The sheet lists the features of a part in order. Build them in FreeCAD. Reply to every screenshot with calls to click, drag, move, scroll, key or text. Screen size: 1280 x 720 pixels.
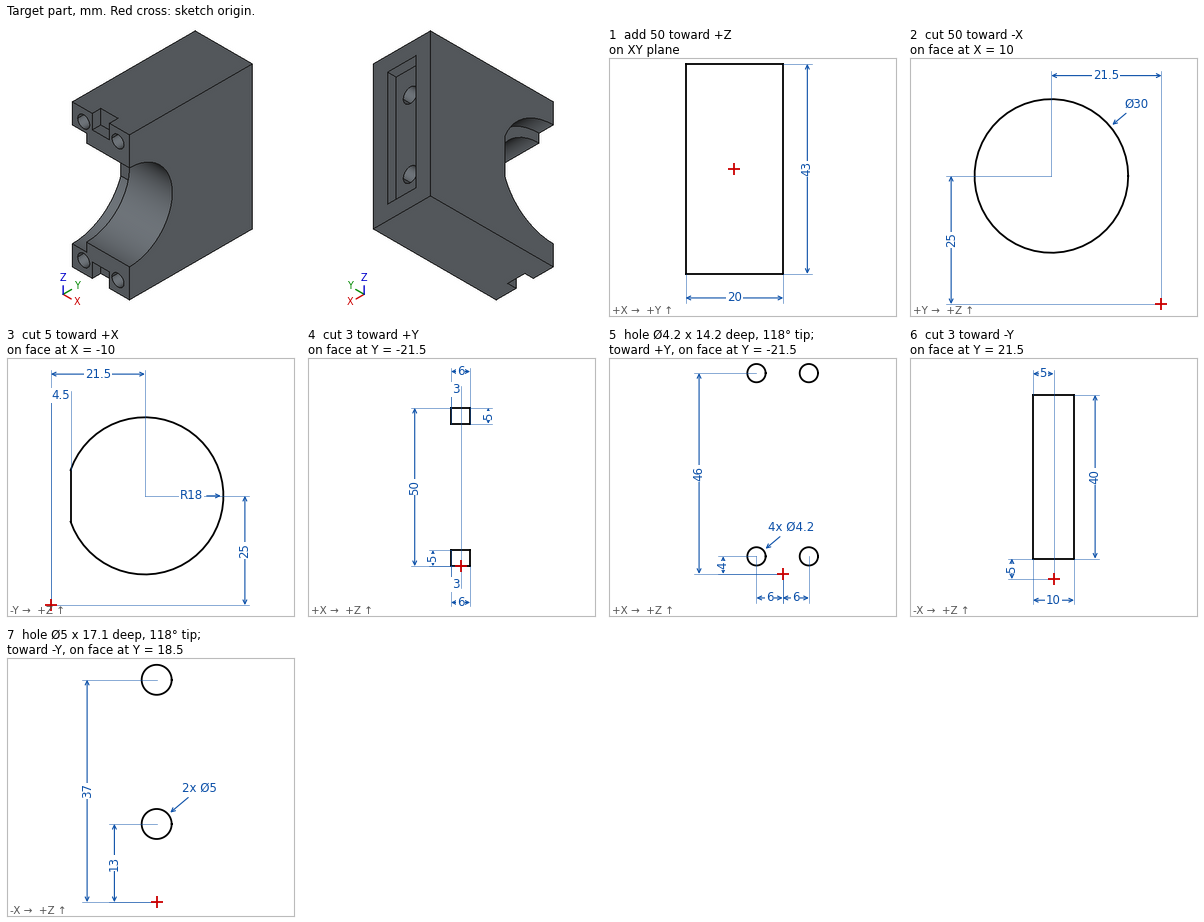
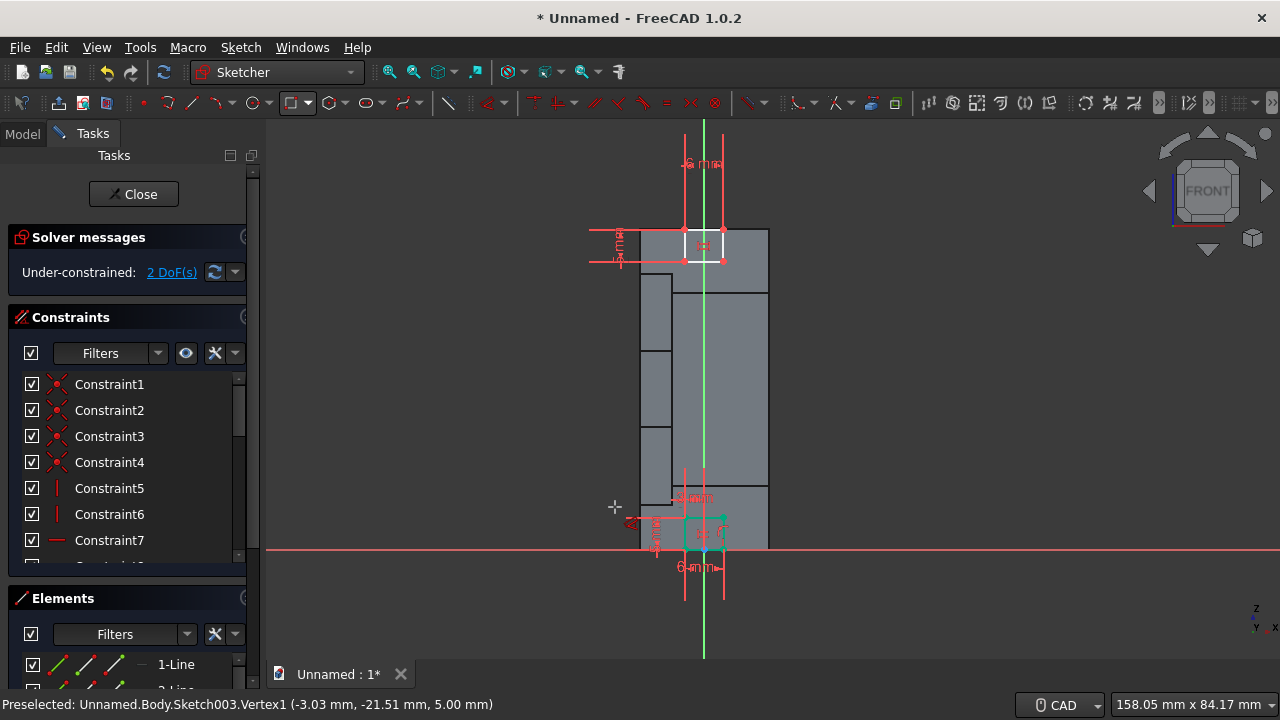
scroll(685, 230, up, 4)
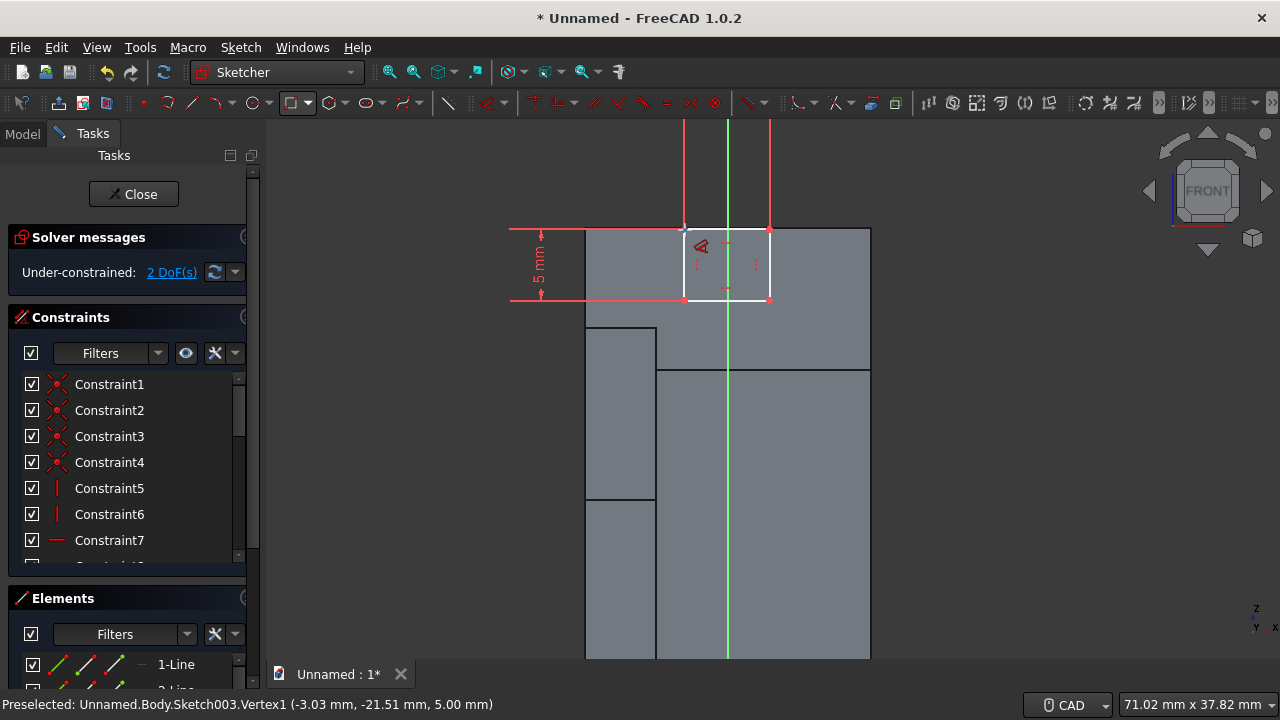
click(684, 229)
click(706, 195)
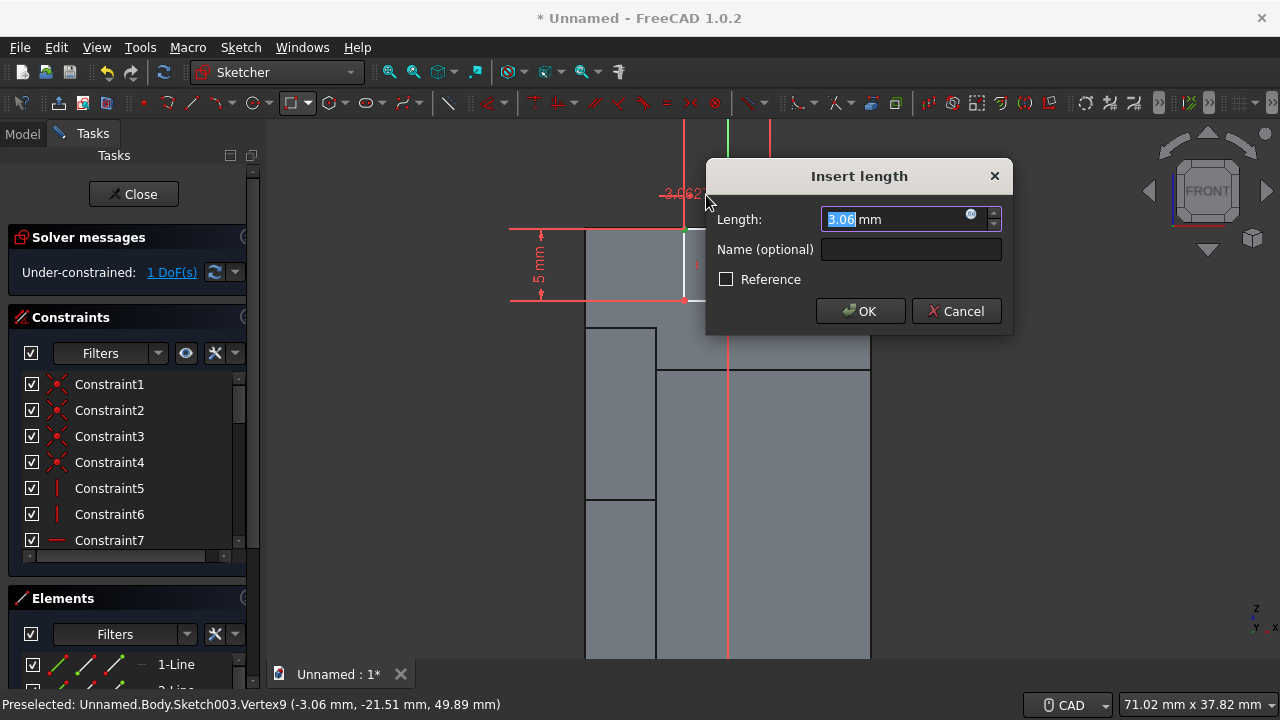
text(3)
key(Return)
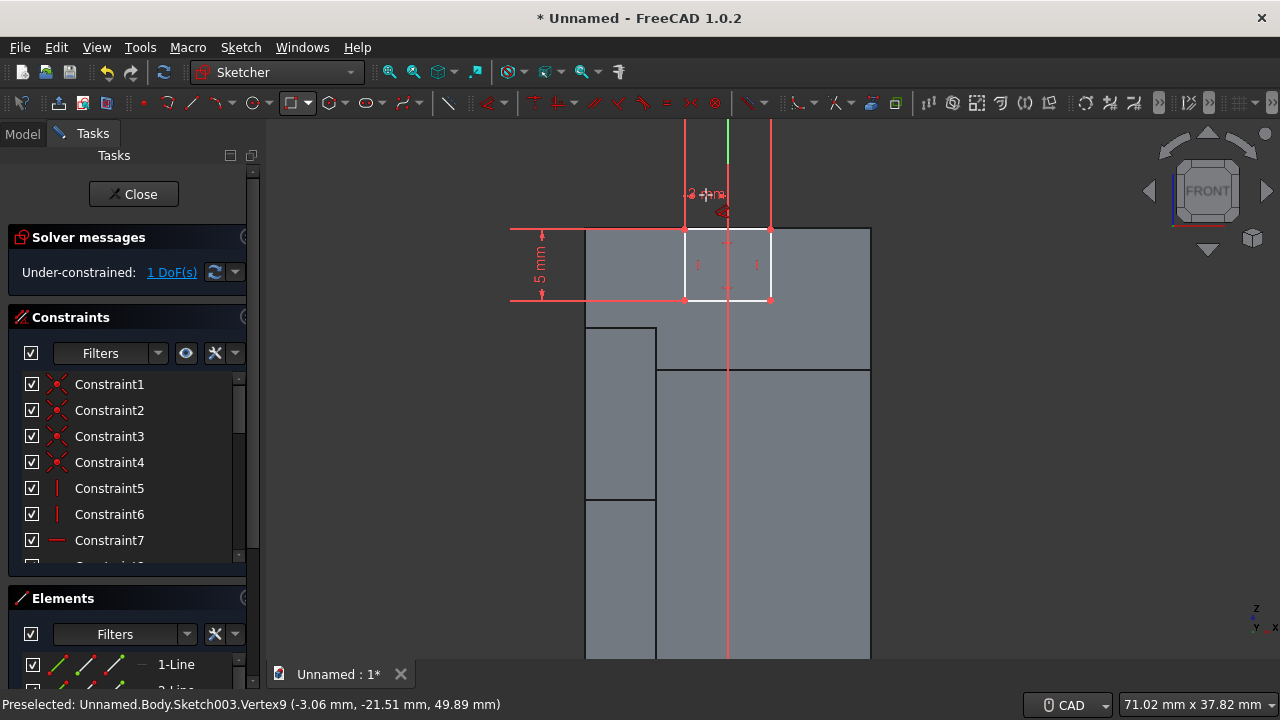
click(685, 229)
click(651, 430)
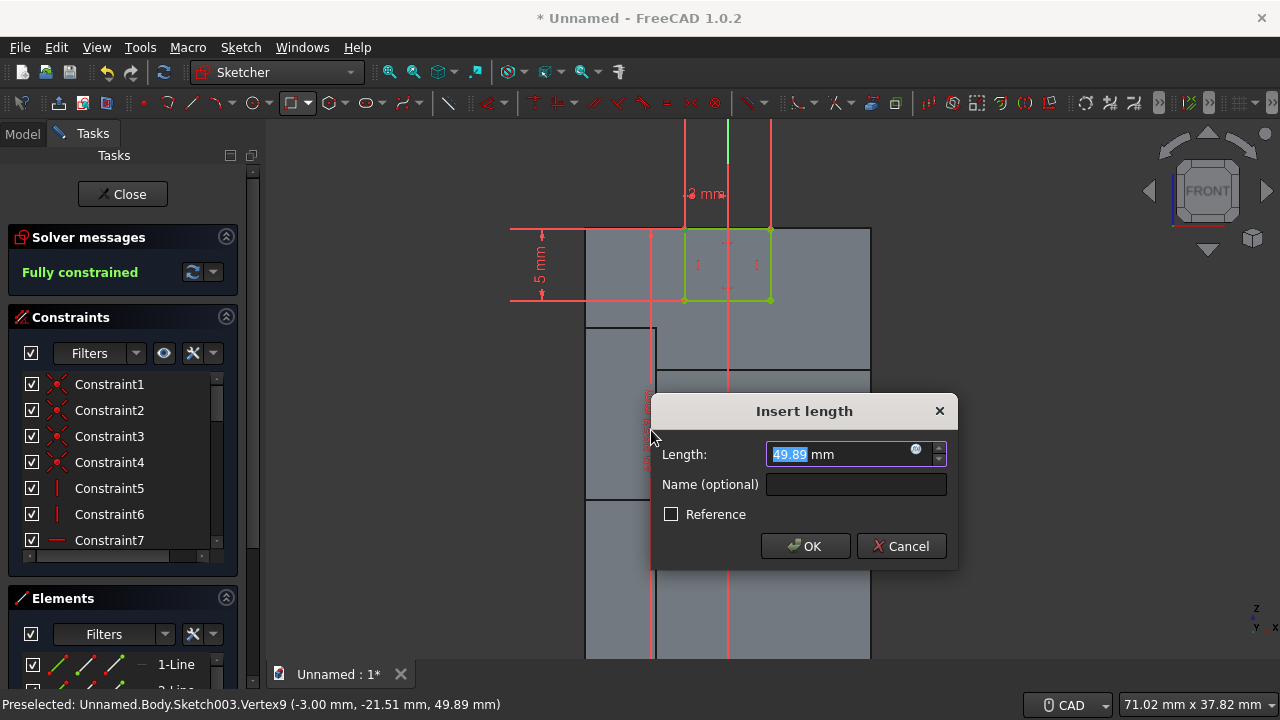
text(50)
key(Return)
key(Escape)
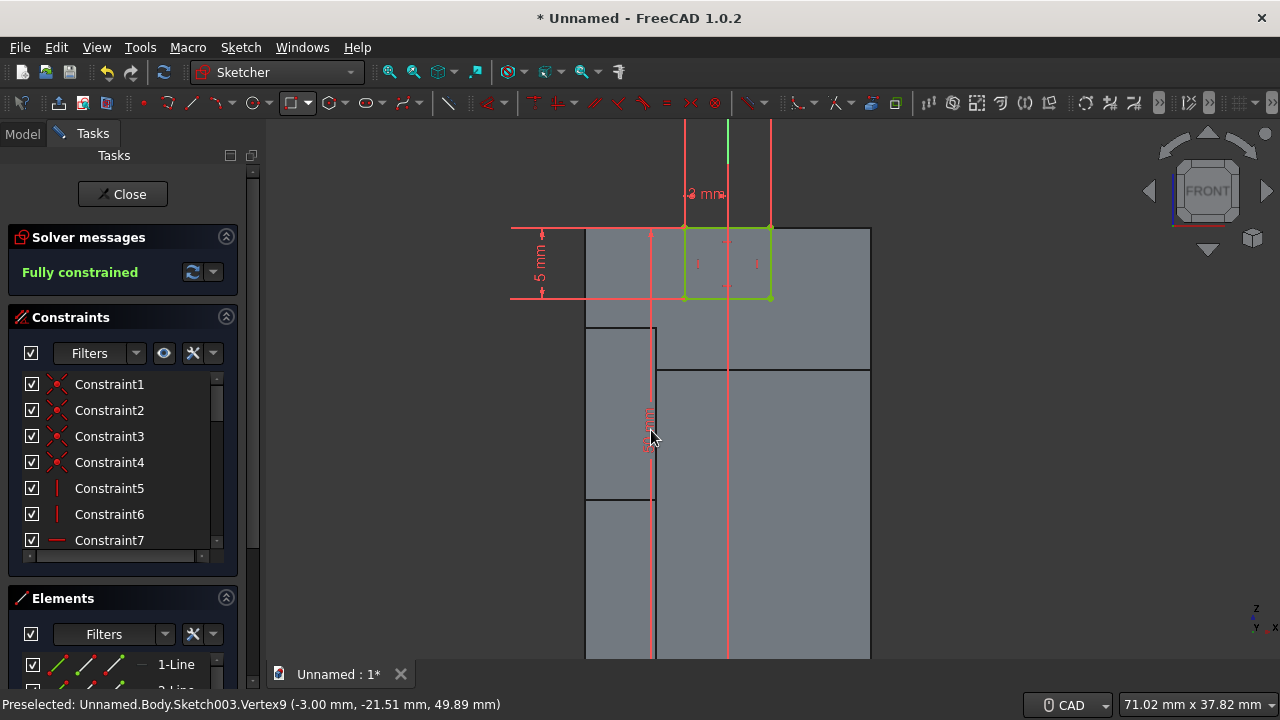
click(123, 194)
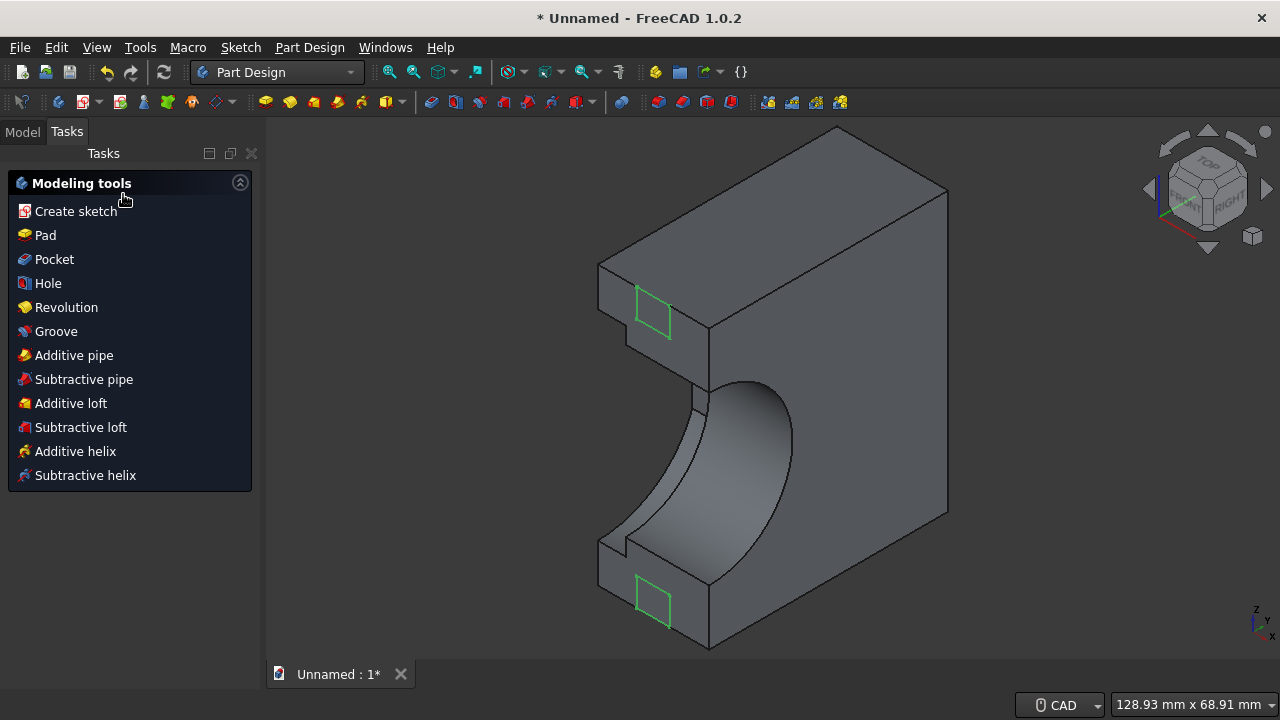
click(432, 102)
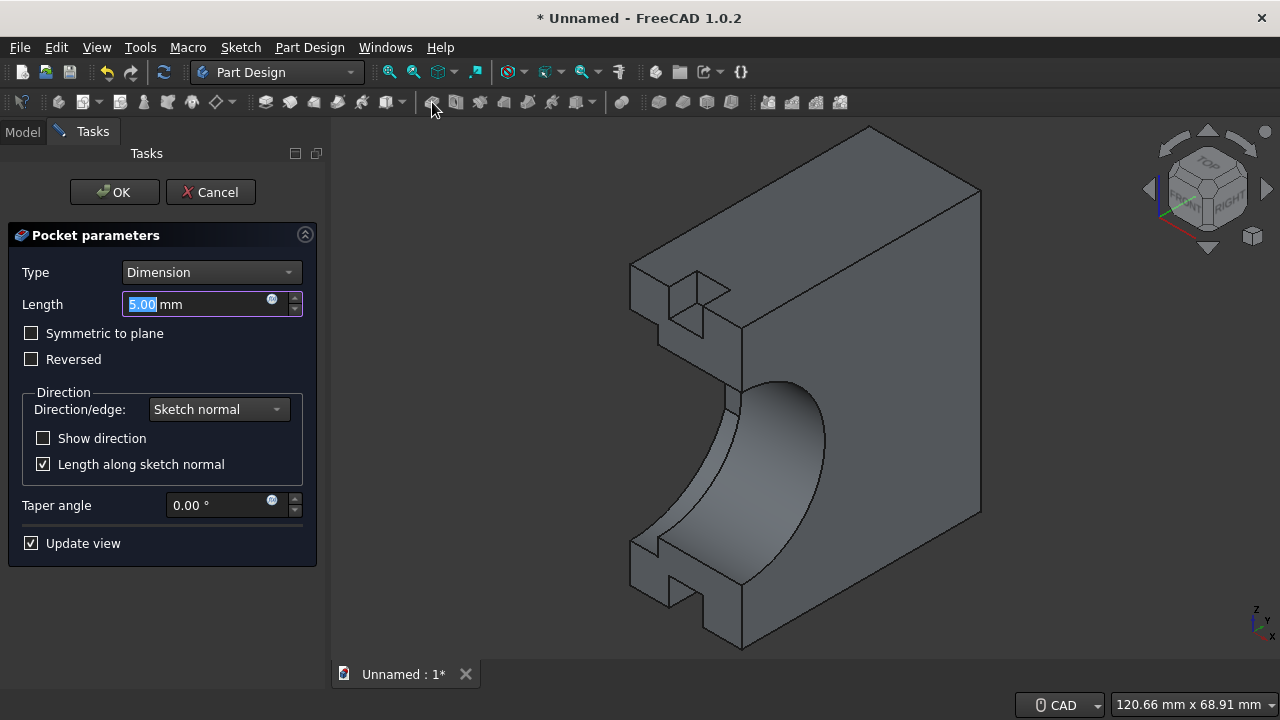
text(3)
key(Tab)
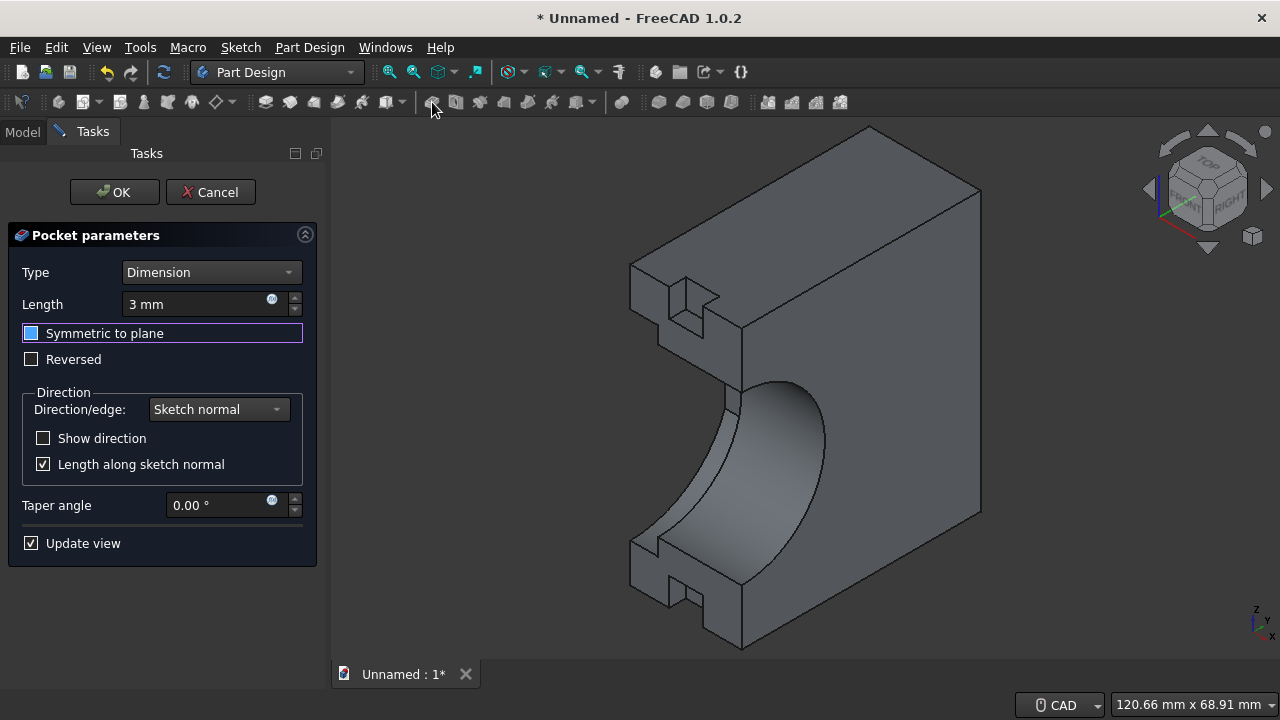
click(115, 192)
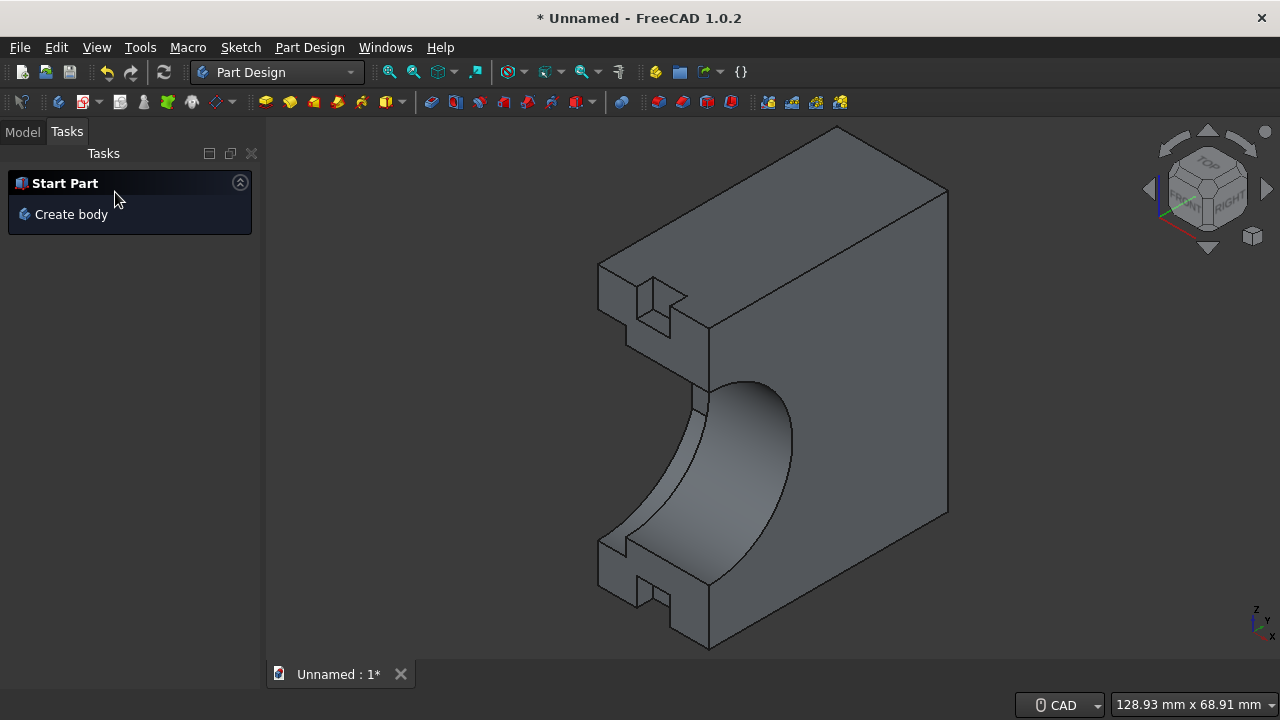
click(685, 355)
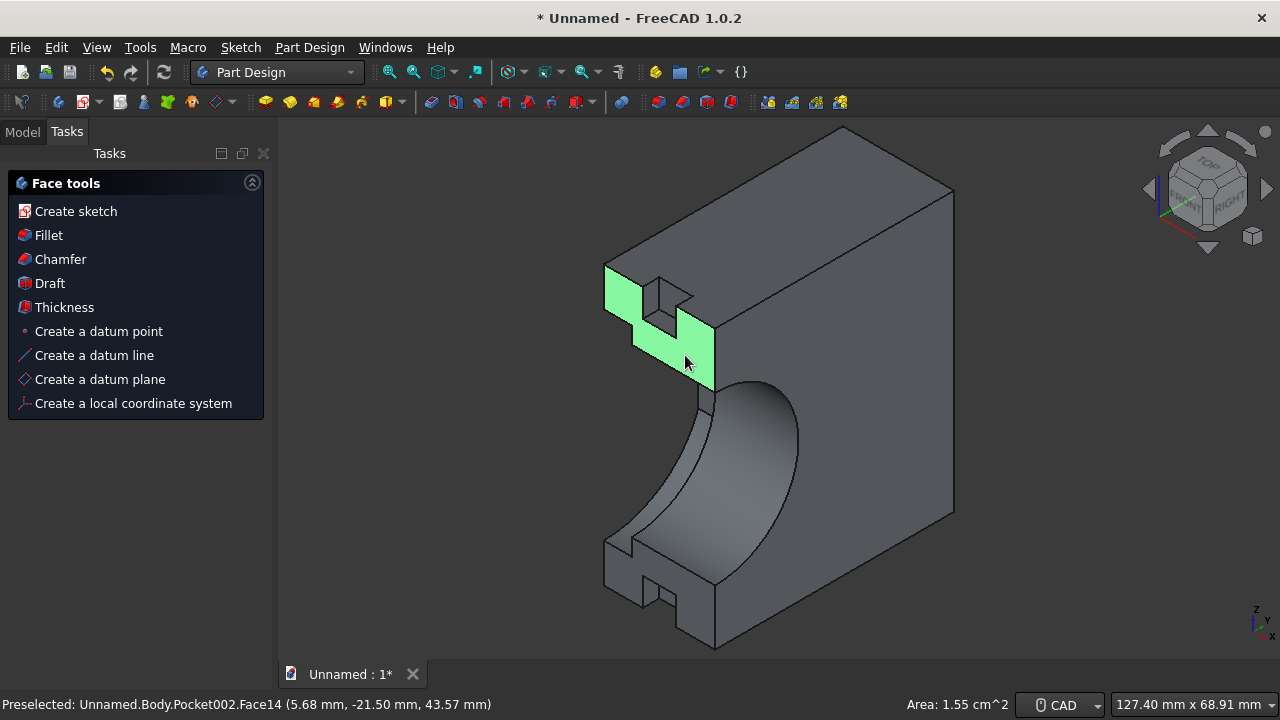
click(84, 102)